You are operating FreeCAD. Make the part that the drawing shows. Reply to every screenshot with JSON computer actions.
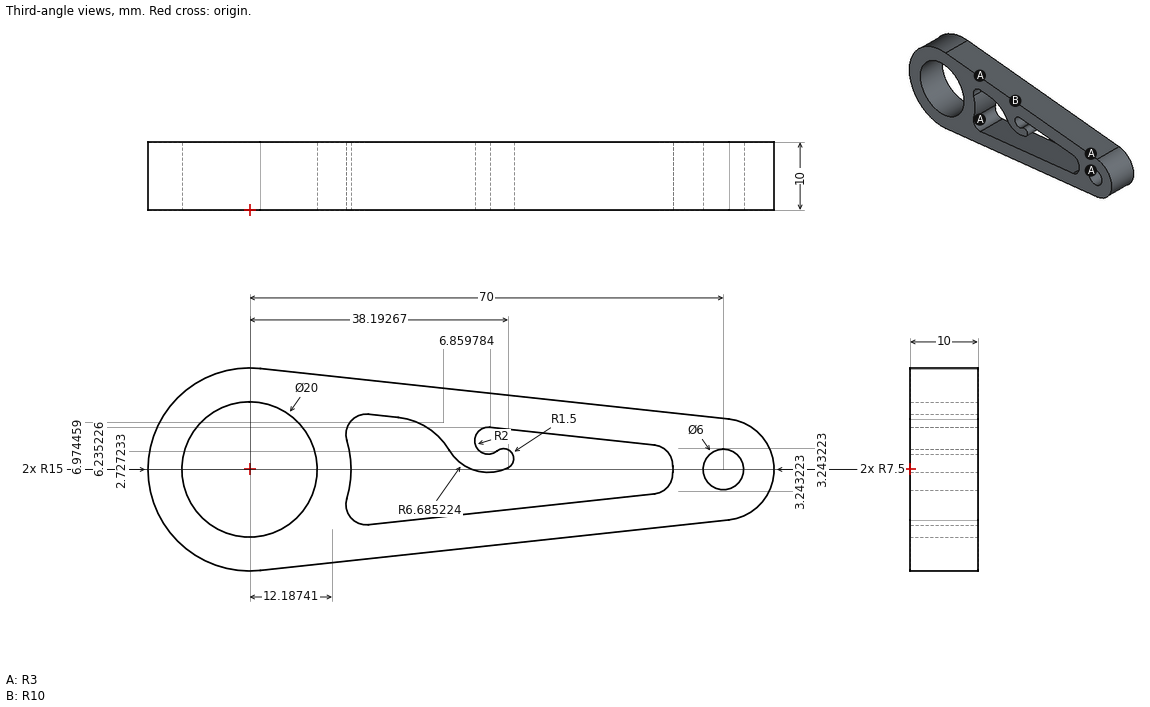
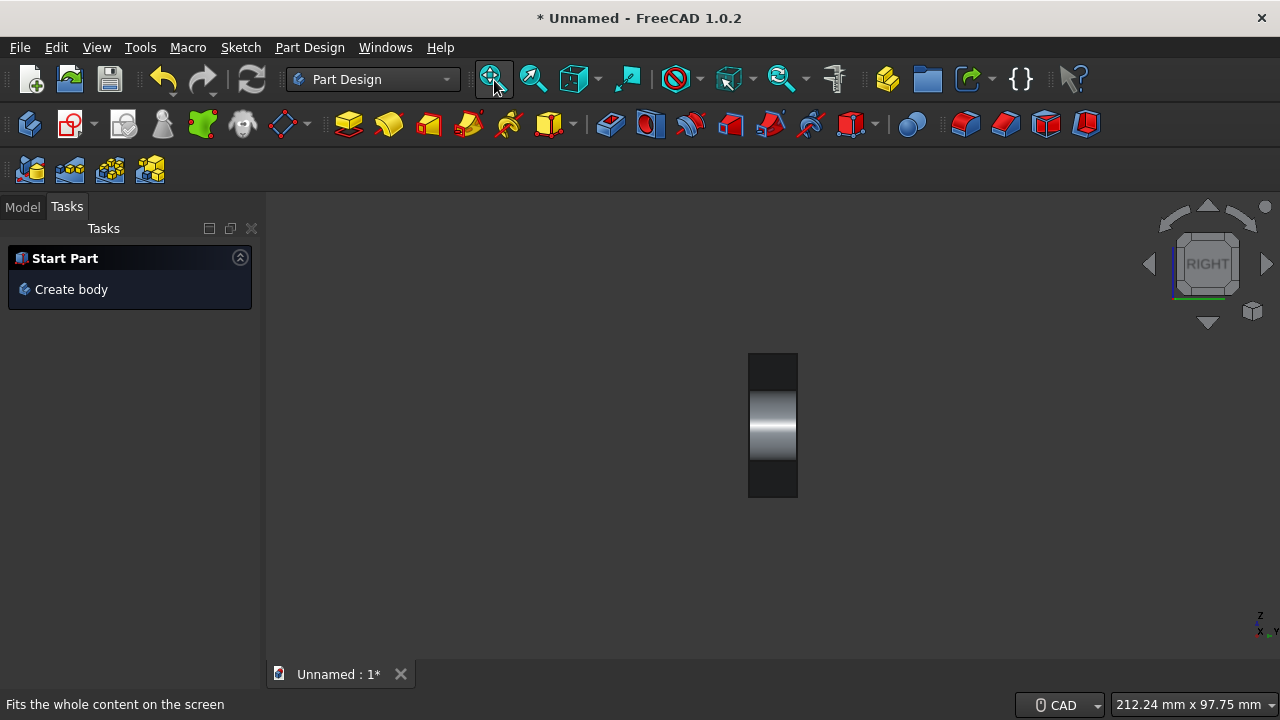
{"action": "key", "text": "5"}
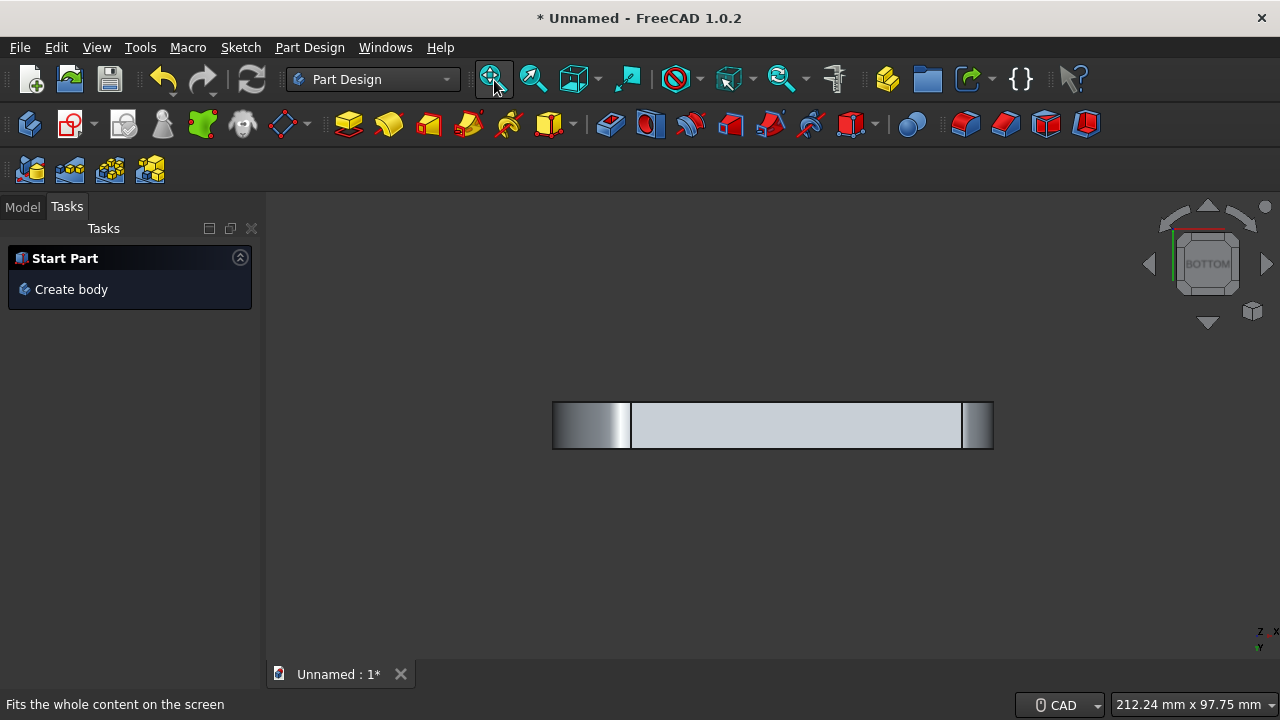
{"action": "left_click", "coordinate": [494, 80]}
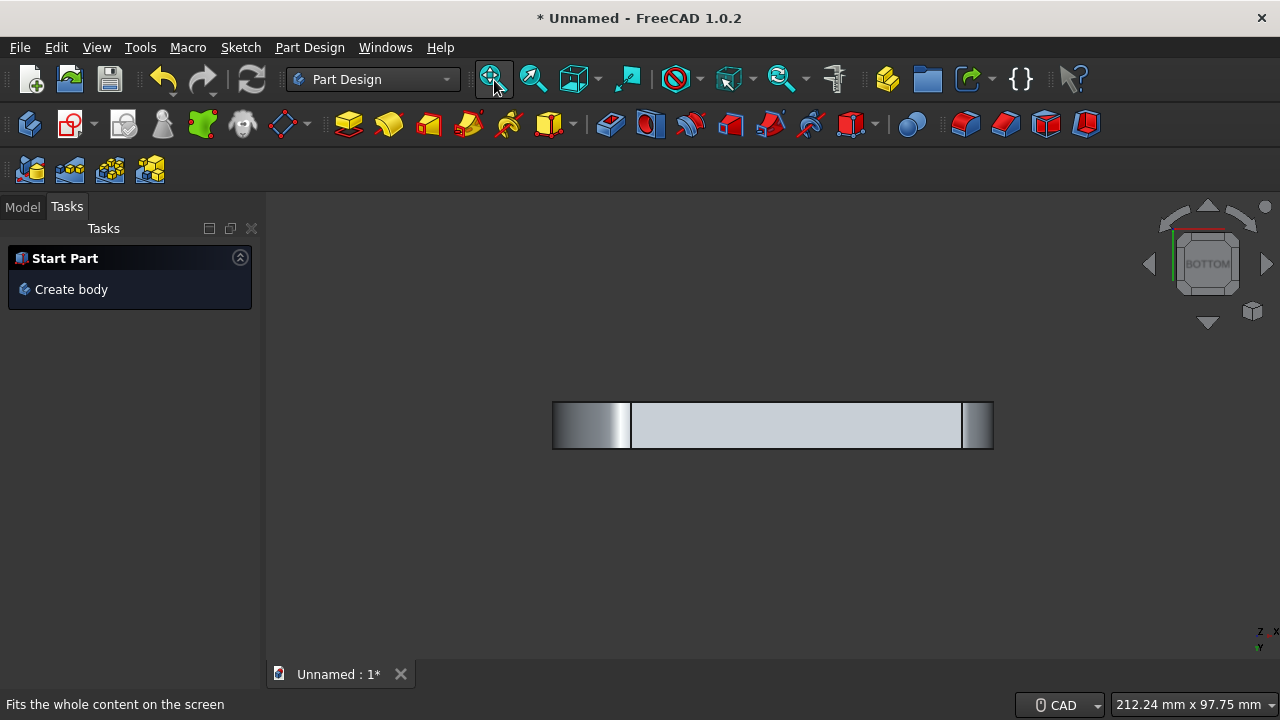
{"action": "key", "text": "4"}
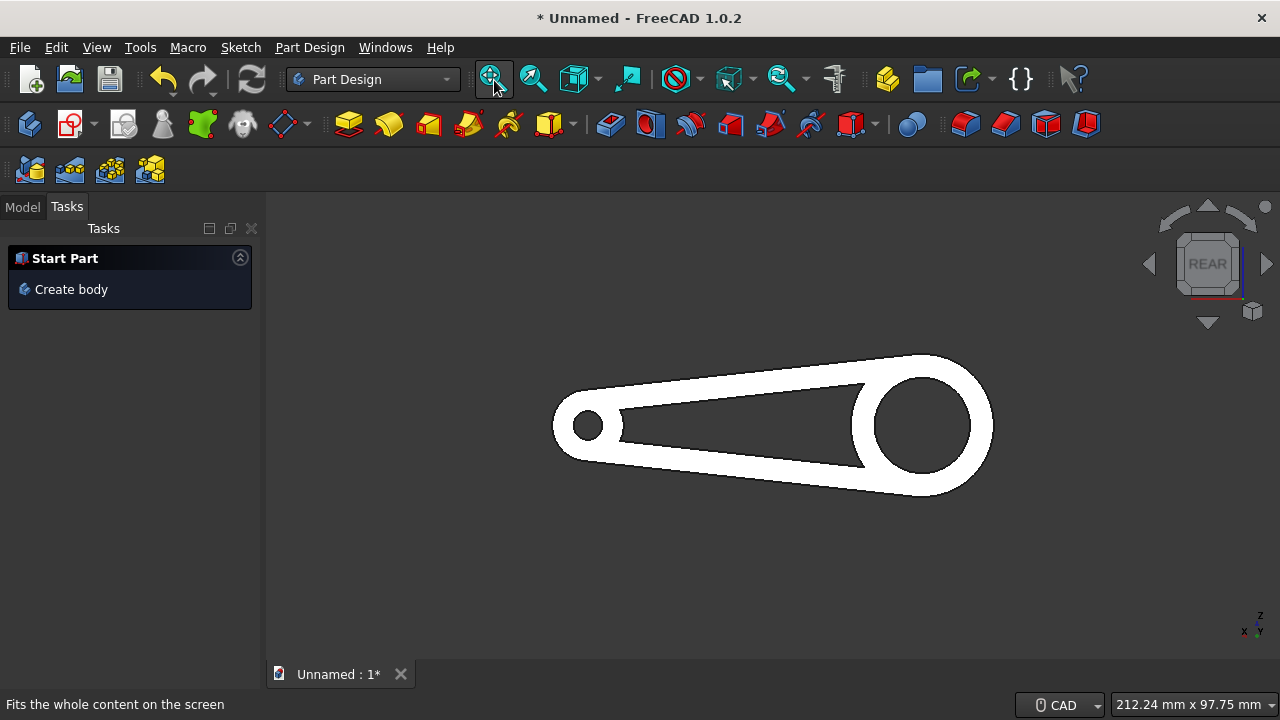
{"action": "left_click", "coordinate": [494, 80]}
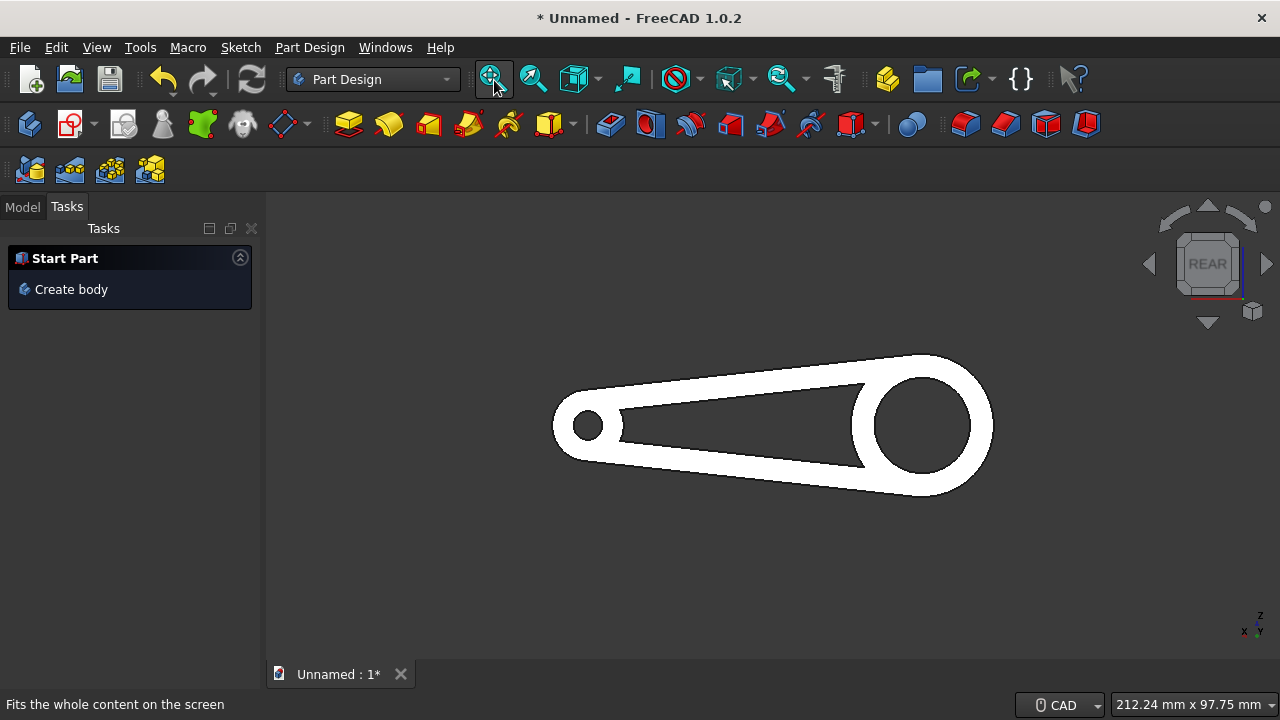
{"action": "key", "text": "6"}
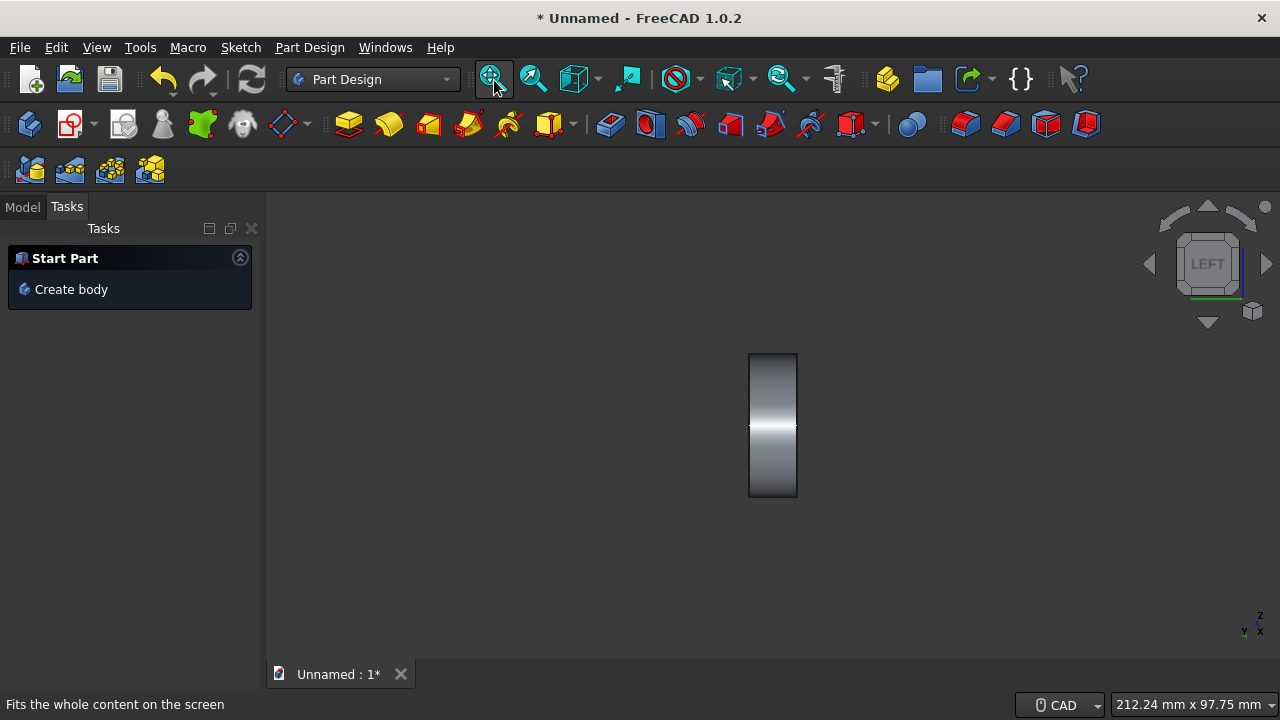
{"action": "left_click", "coordinate": [494, 80]}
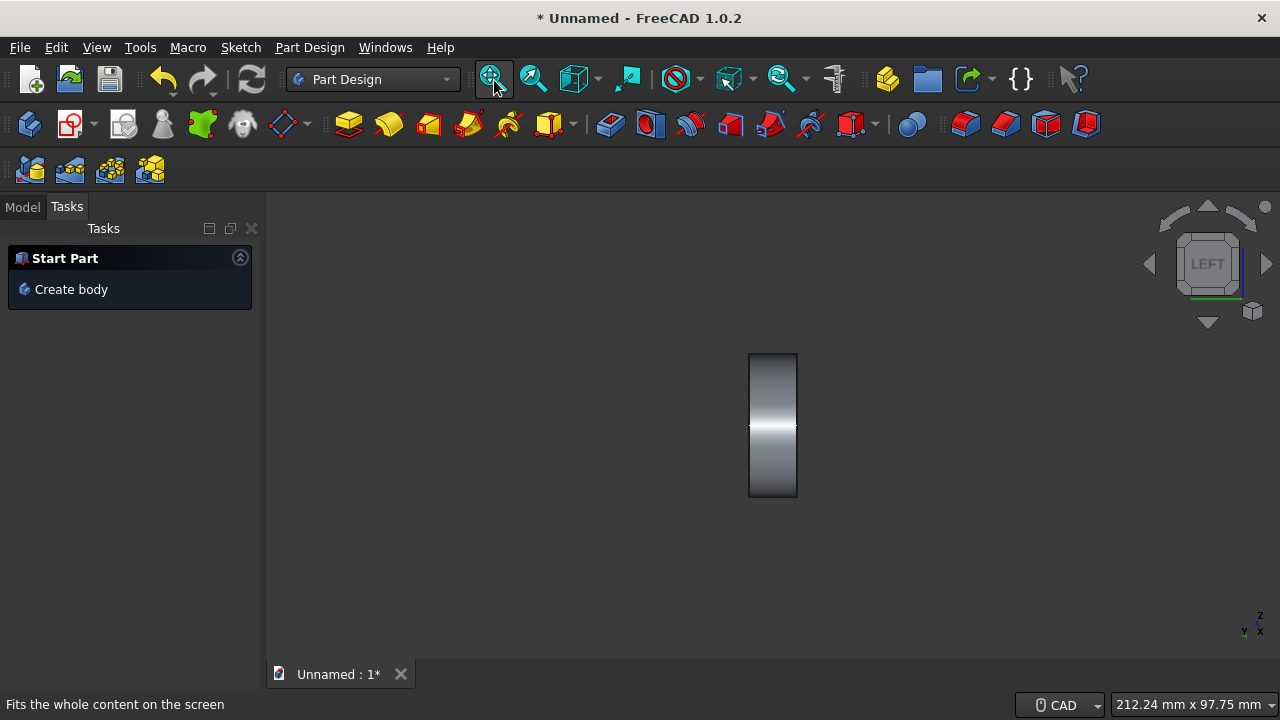
{"action": "key", "text": "v 3"}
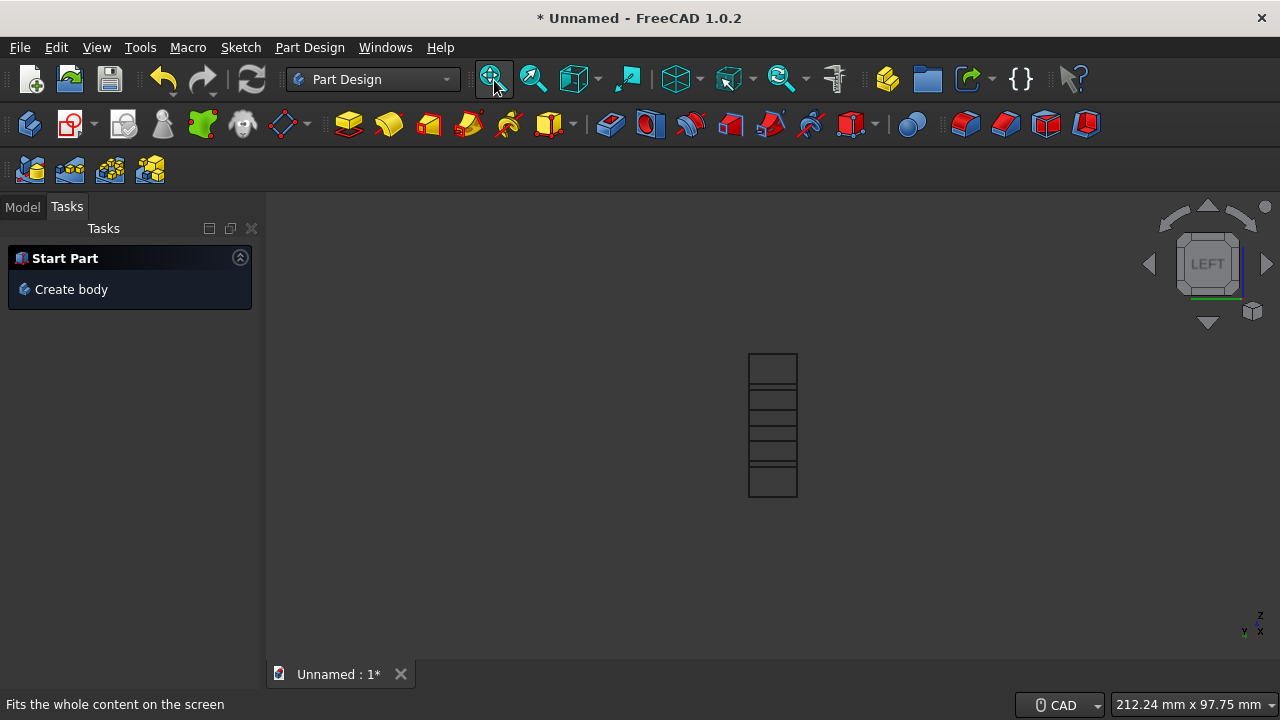
{"action": "key", "text": "0"}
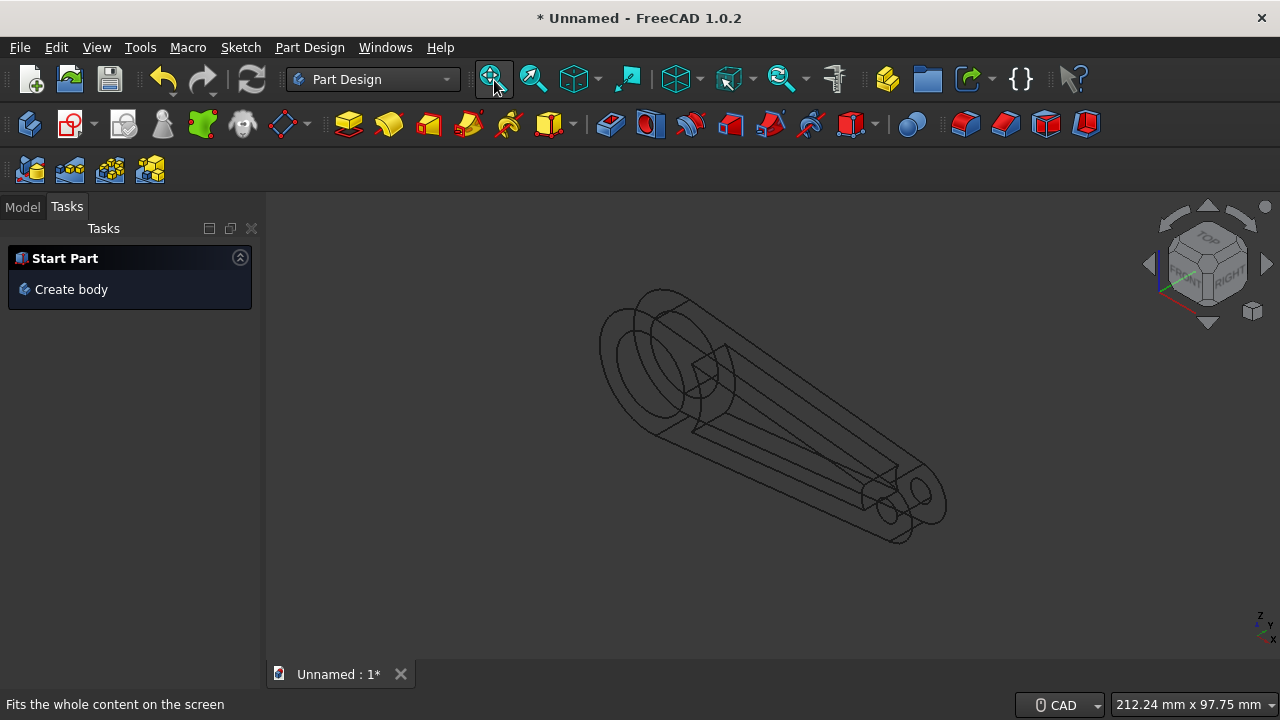
{"action": "left_click", "coordinate": [709, 421]}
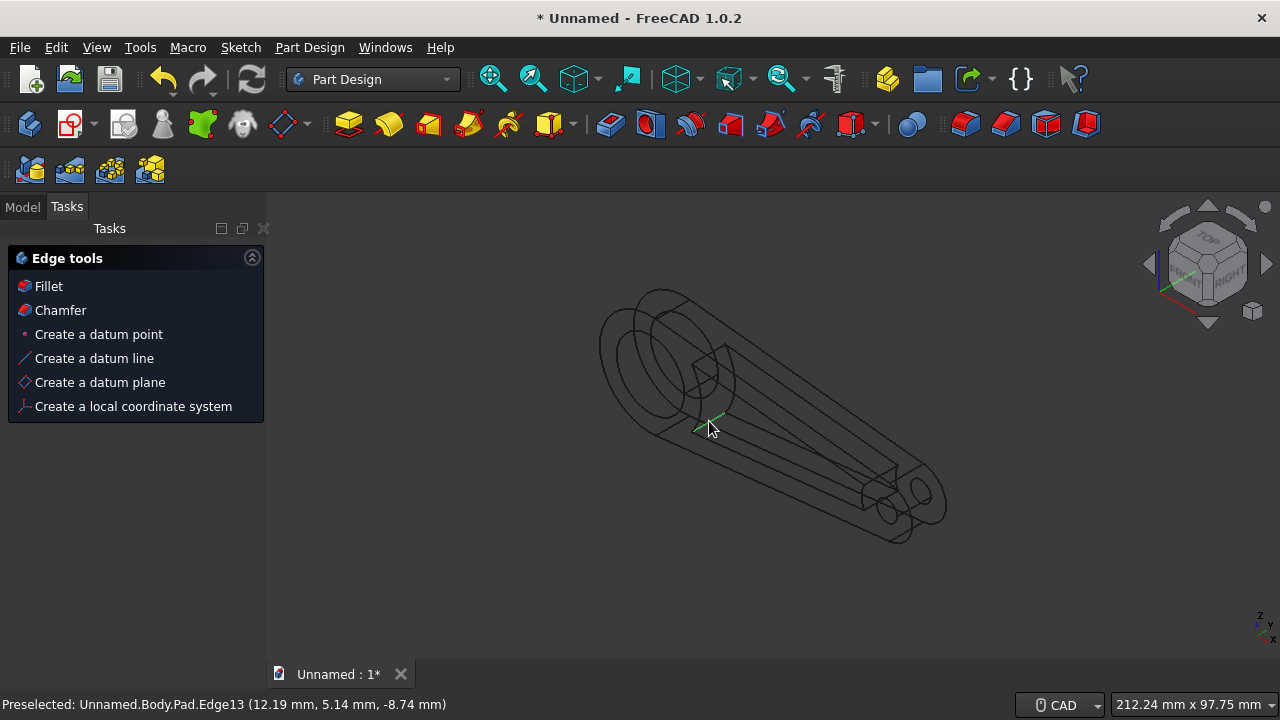
{"action": "left_click", "coordinate": [721, 349], "text": "ctrl"}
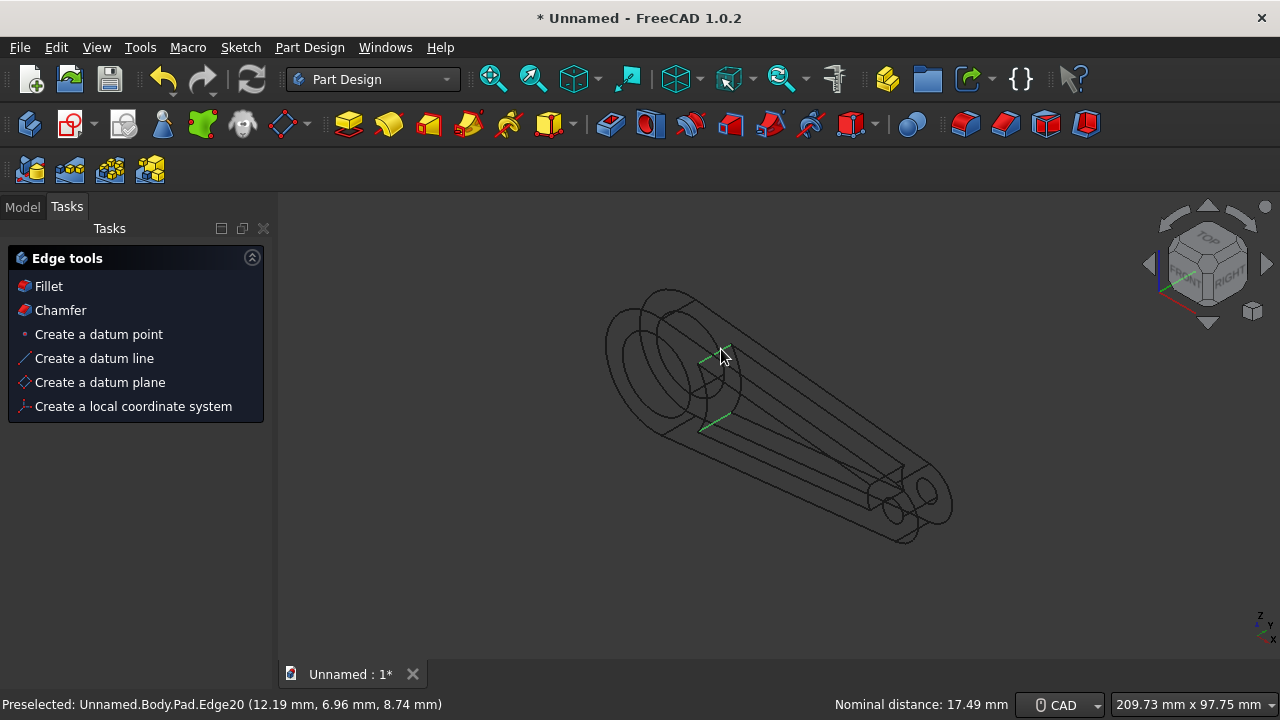
{"action": "left_click", "coordinate": [894, 470], "text": "ctrl"}